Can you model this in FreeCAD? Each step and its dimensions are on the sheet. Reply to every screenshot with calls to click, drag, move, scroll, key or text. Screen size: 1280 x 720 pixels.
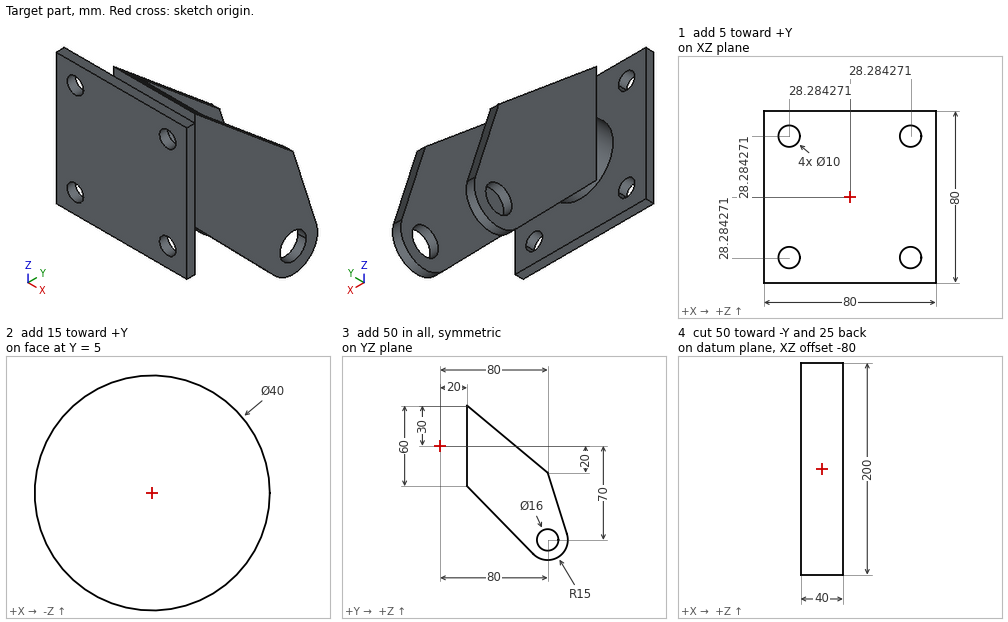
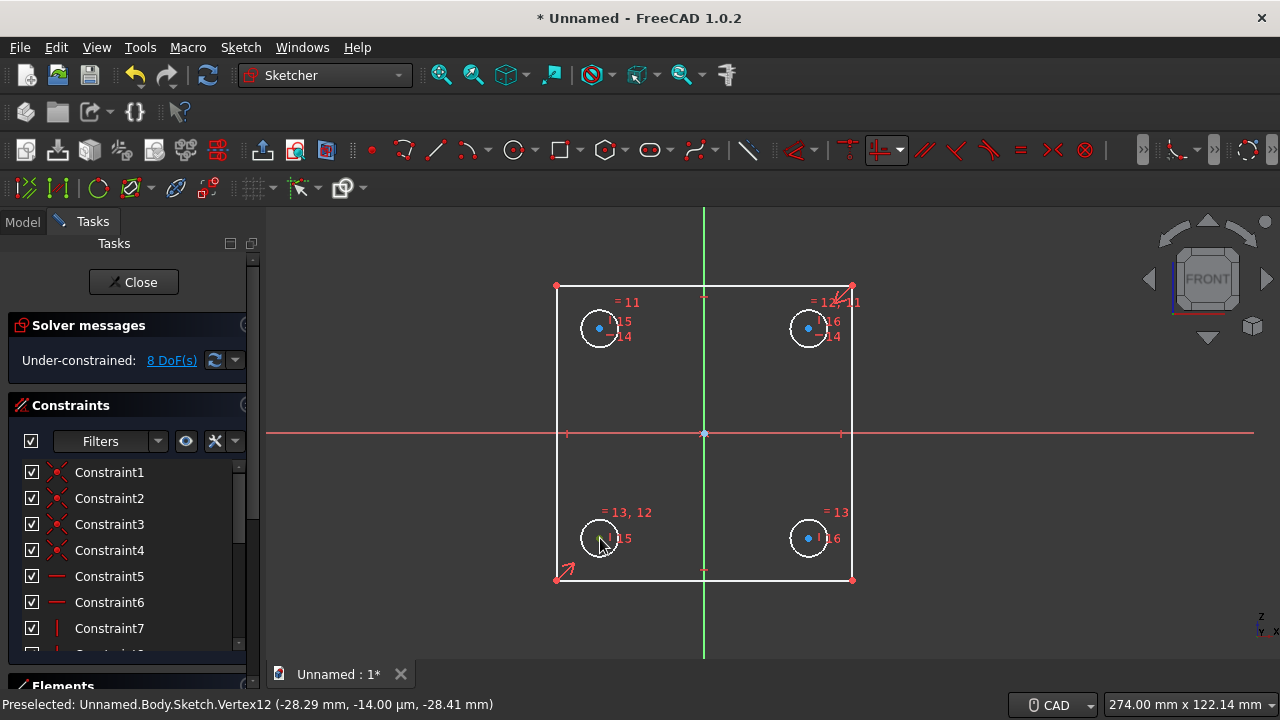
click(809, 538)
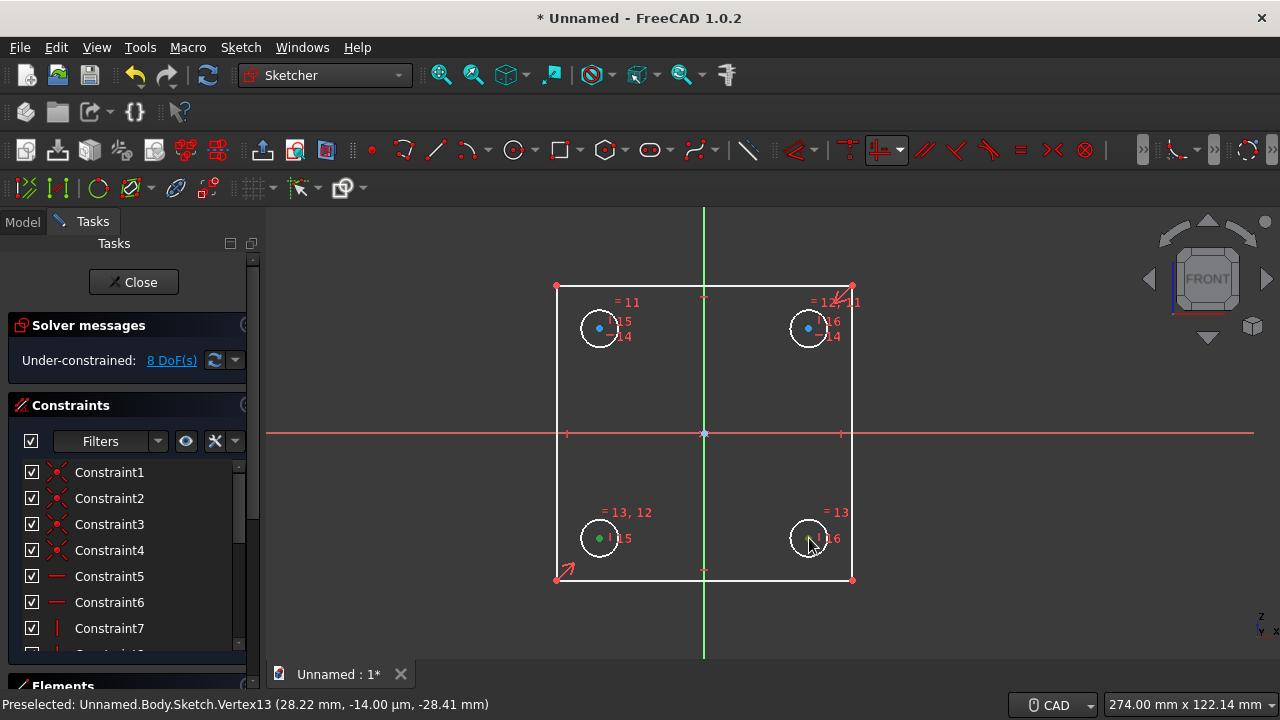
click(902, 150)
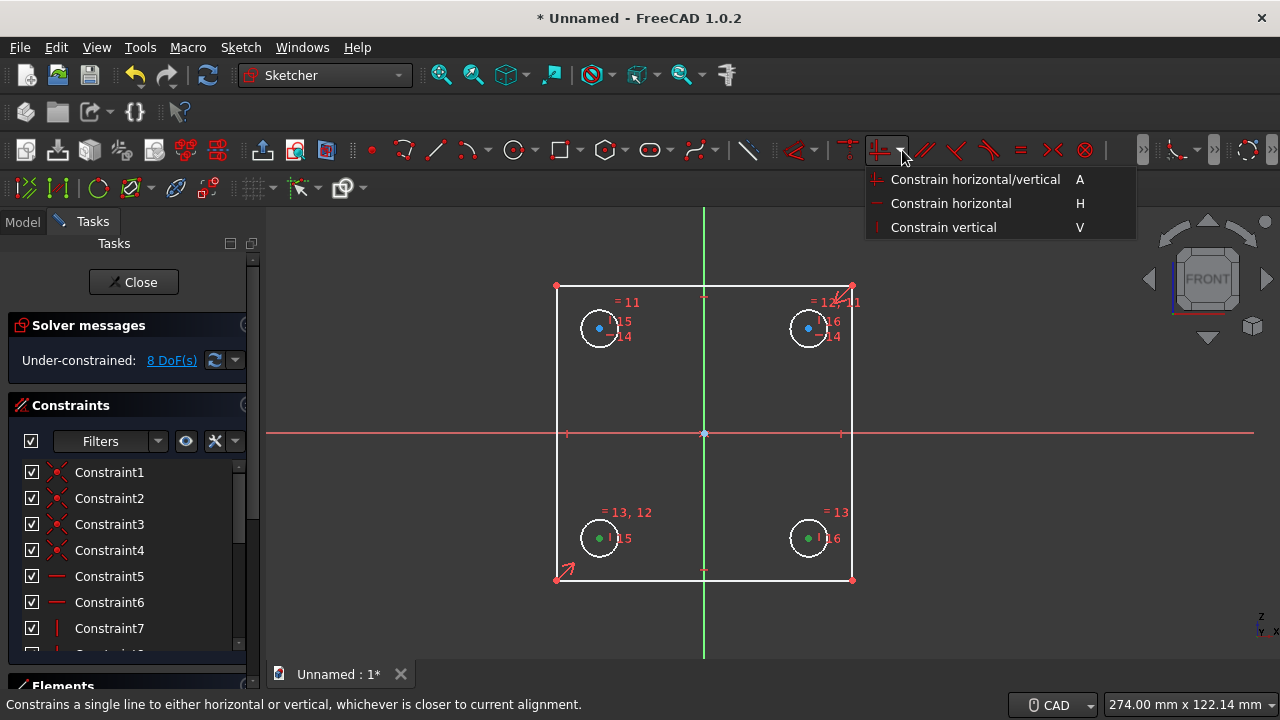
click(1001, 203)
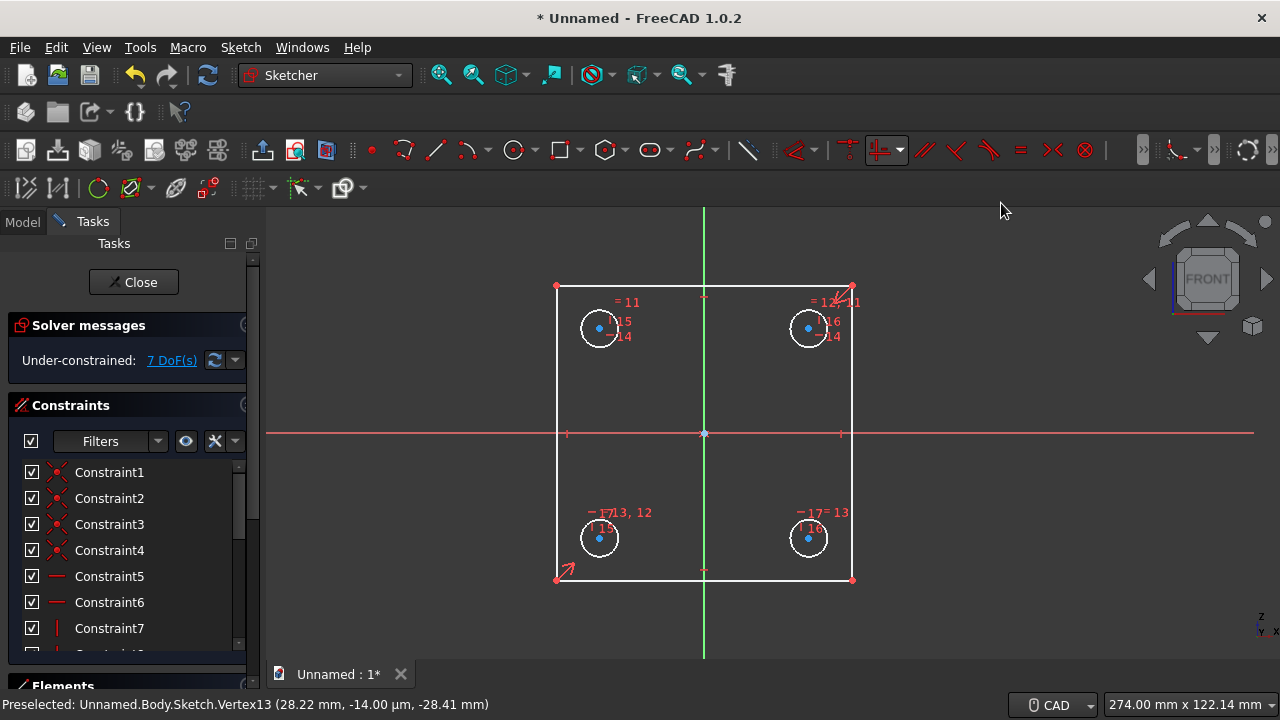
click(794, 150)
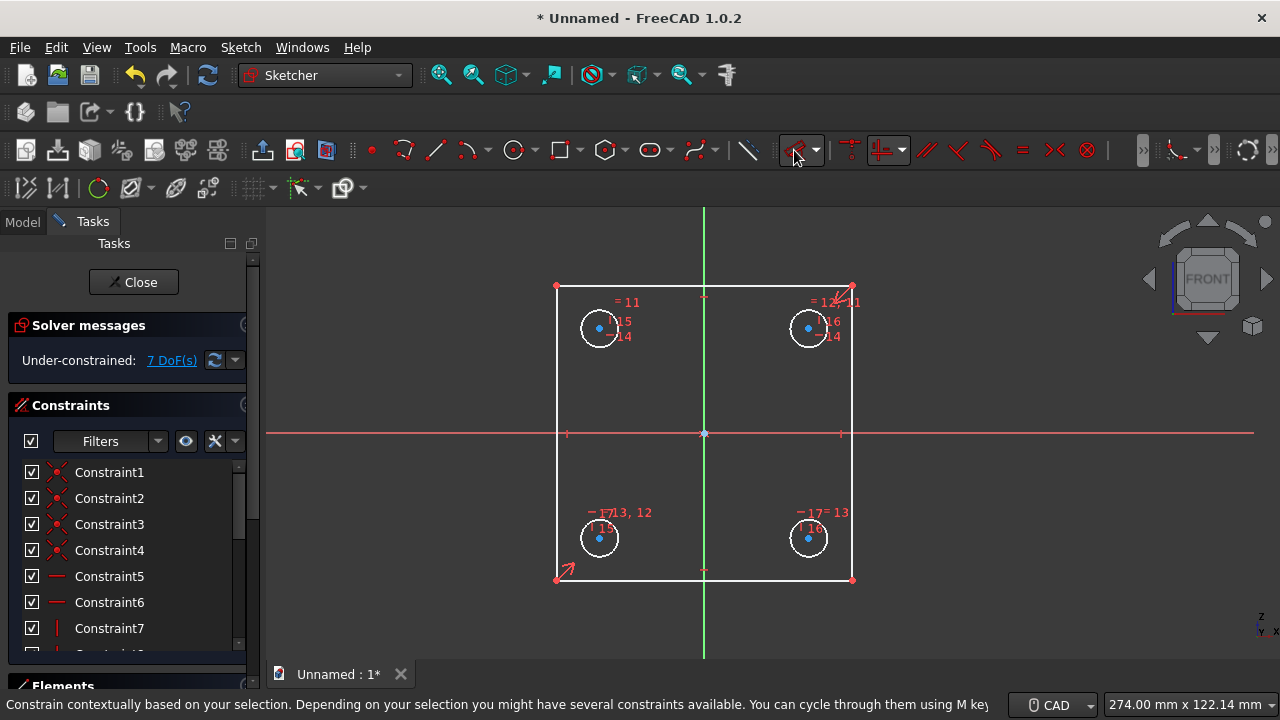
click(613, 316)
click(648, 315)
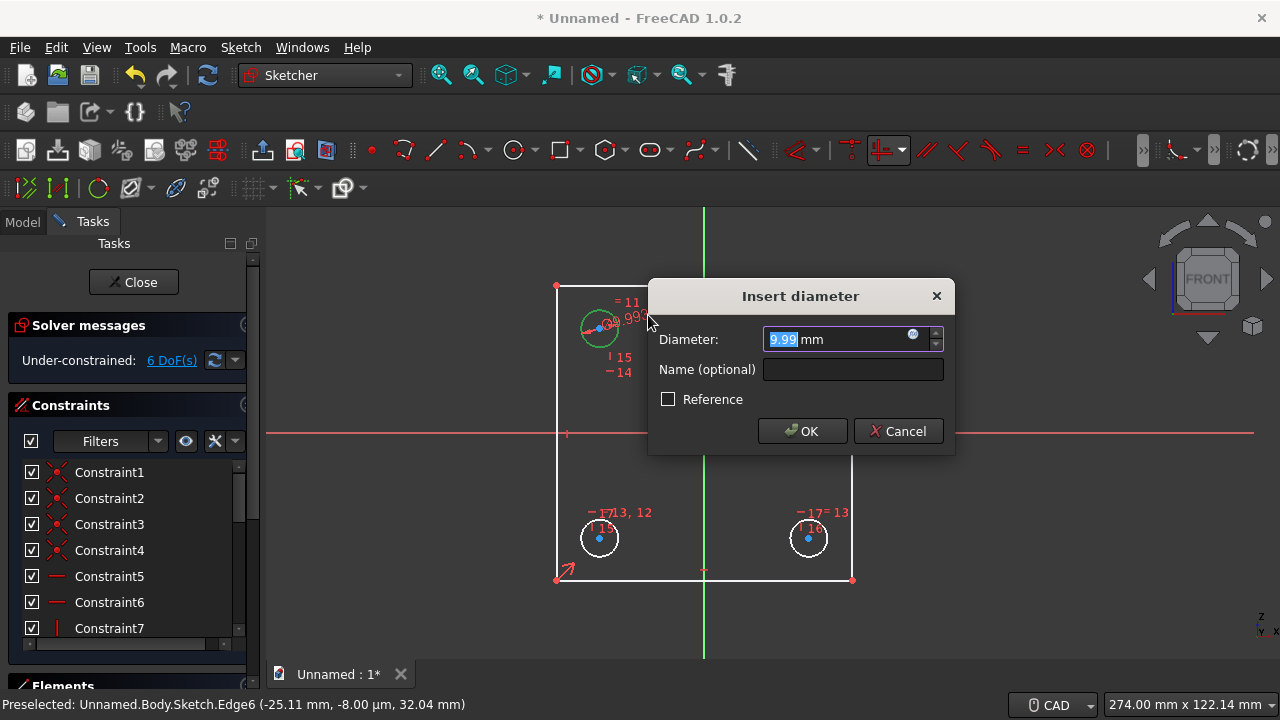
text(10)
key(Return)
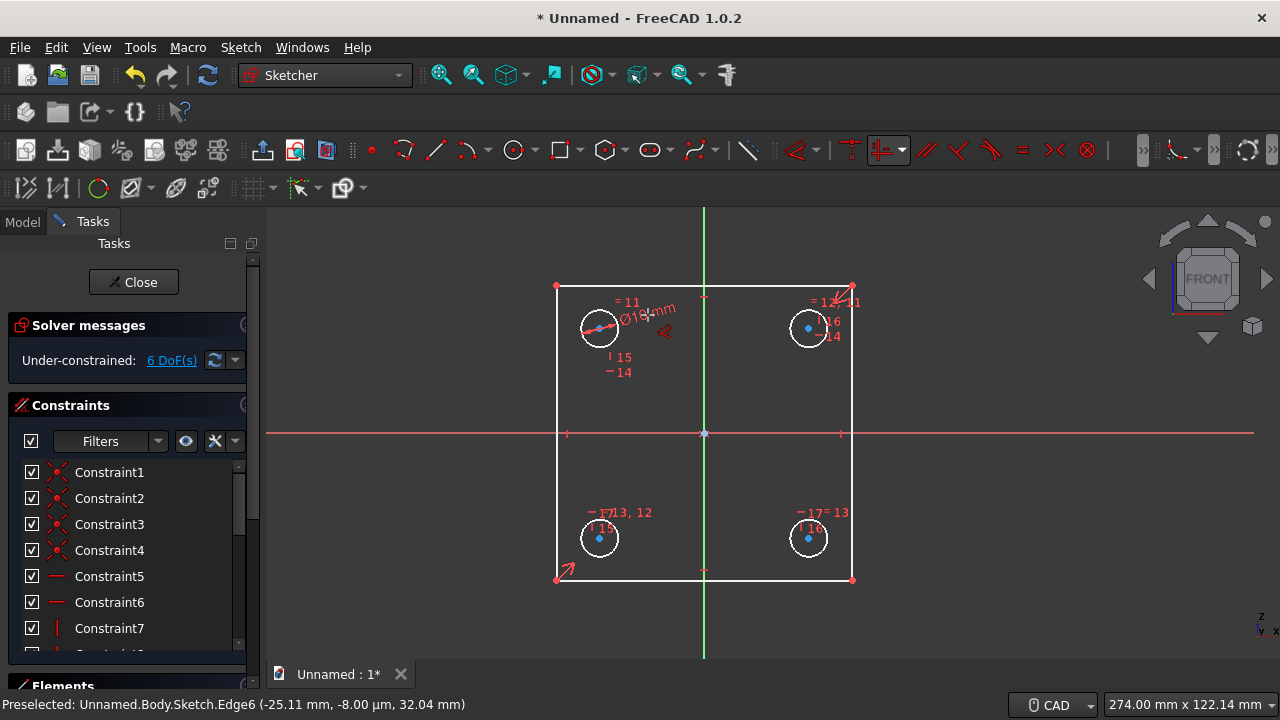
click(645, 581)
click(636, 615)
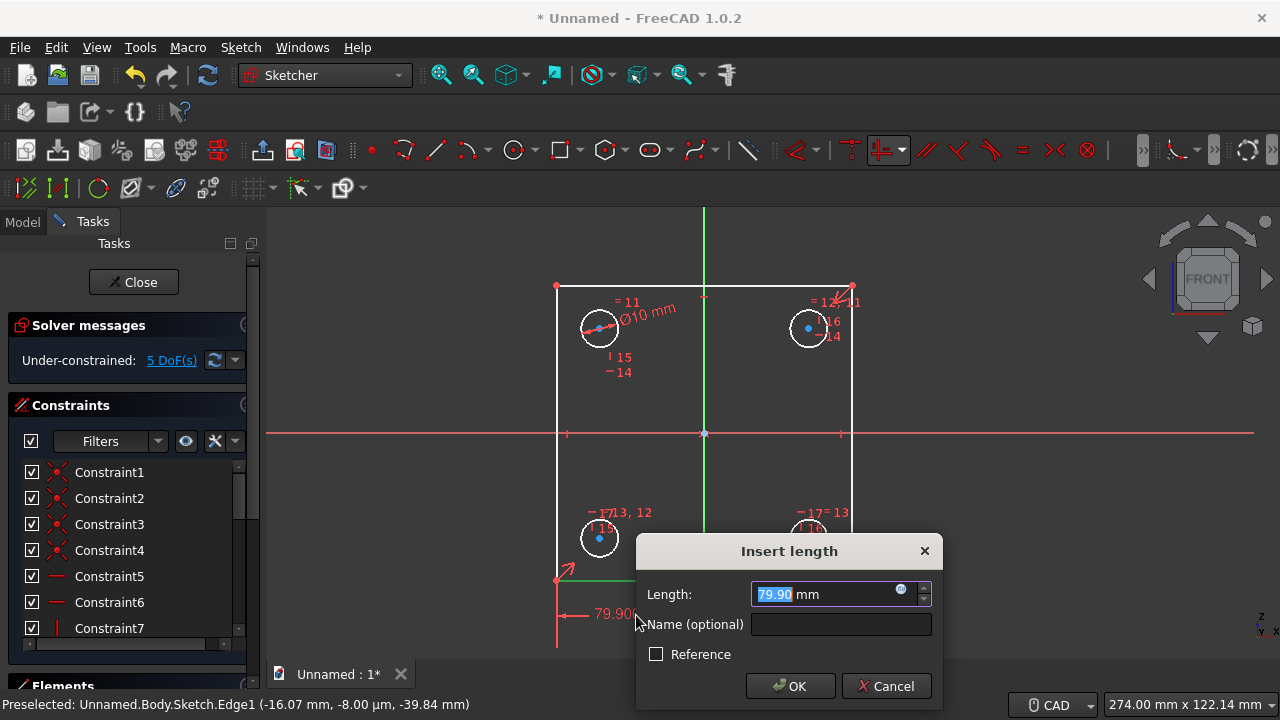
text(80)
key(Return)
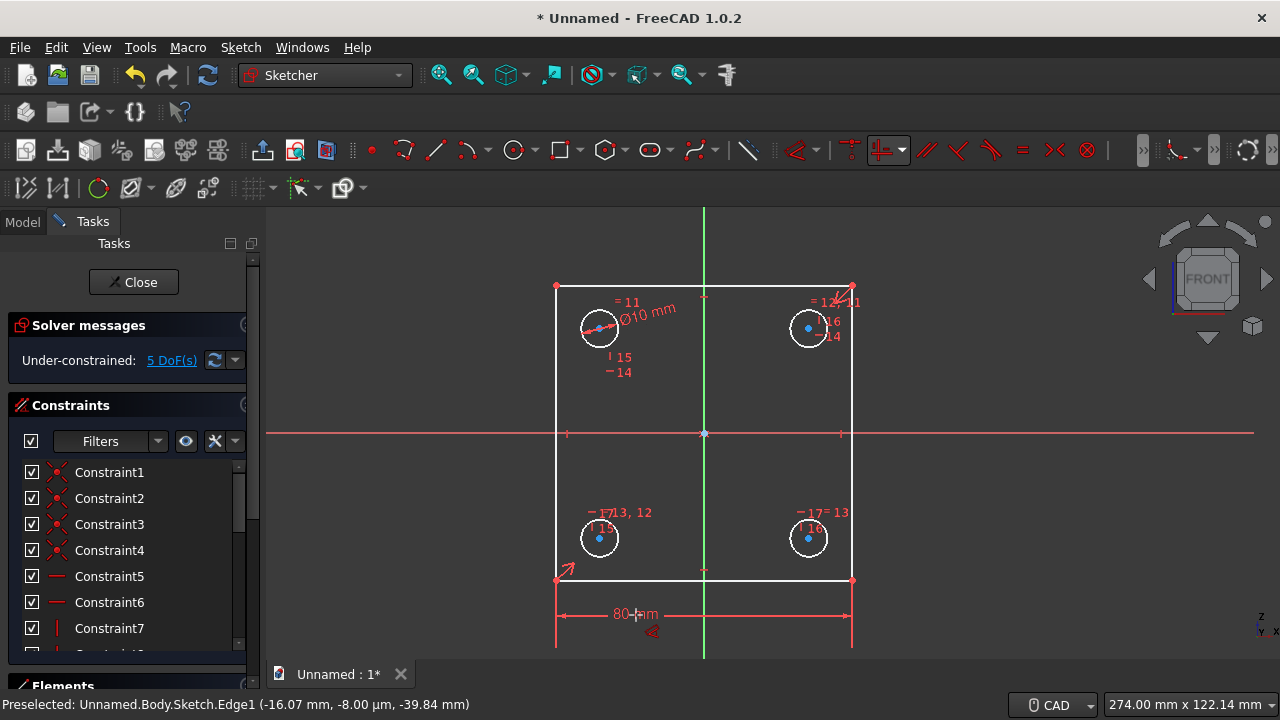
click(853, 492)
click(887, 365)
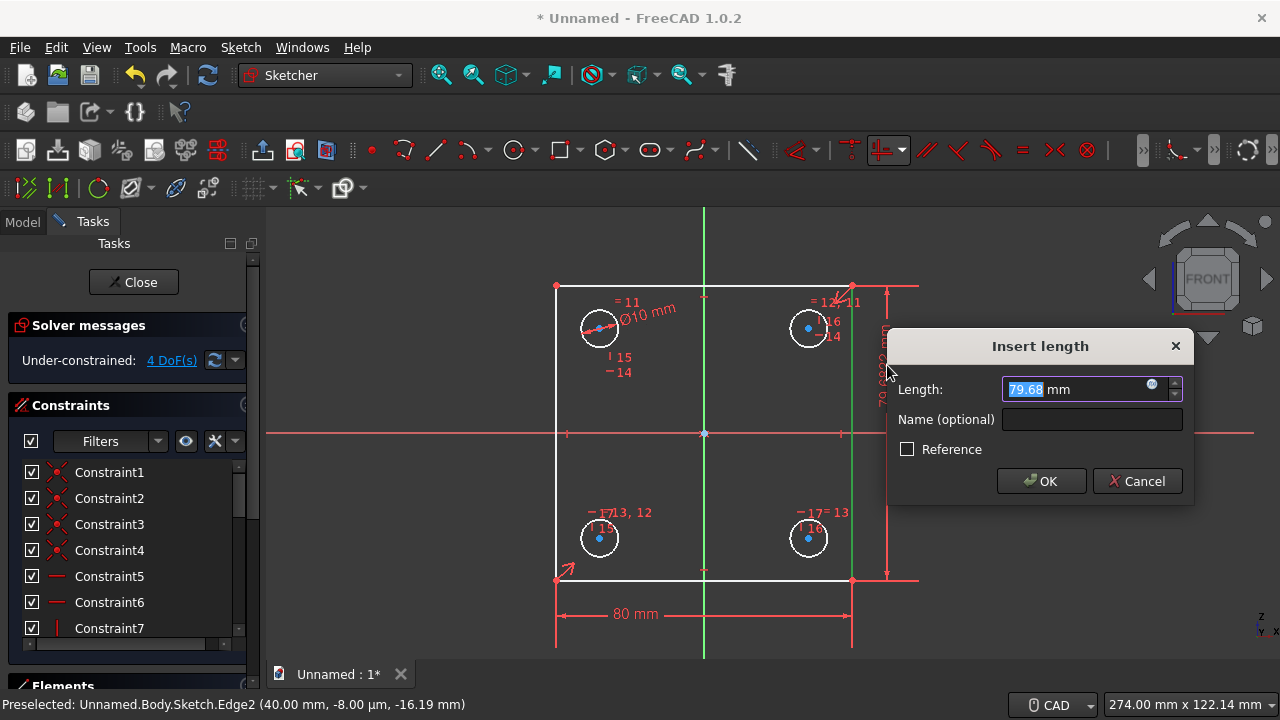
text(80)
key(Return)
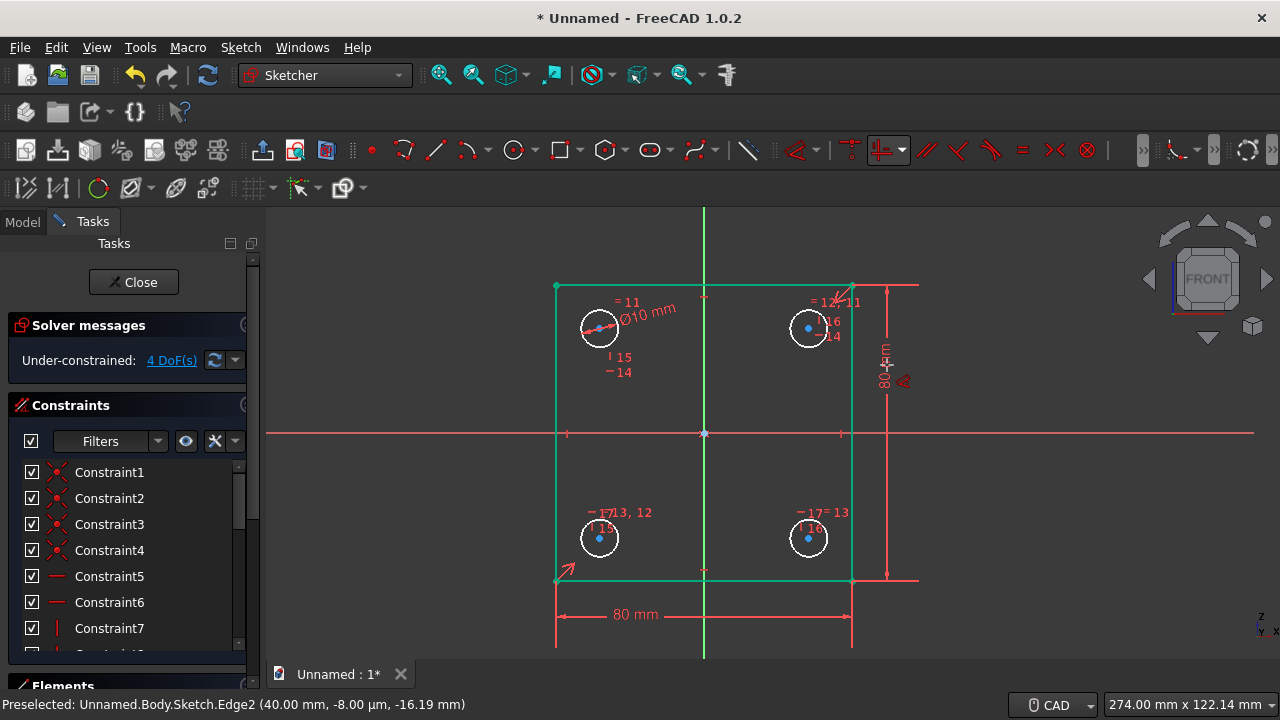
click(600, 329)
click(652, 467)